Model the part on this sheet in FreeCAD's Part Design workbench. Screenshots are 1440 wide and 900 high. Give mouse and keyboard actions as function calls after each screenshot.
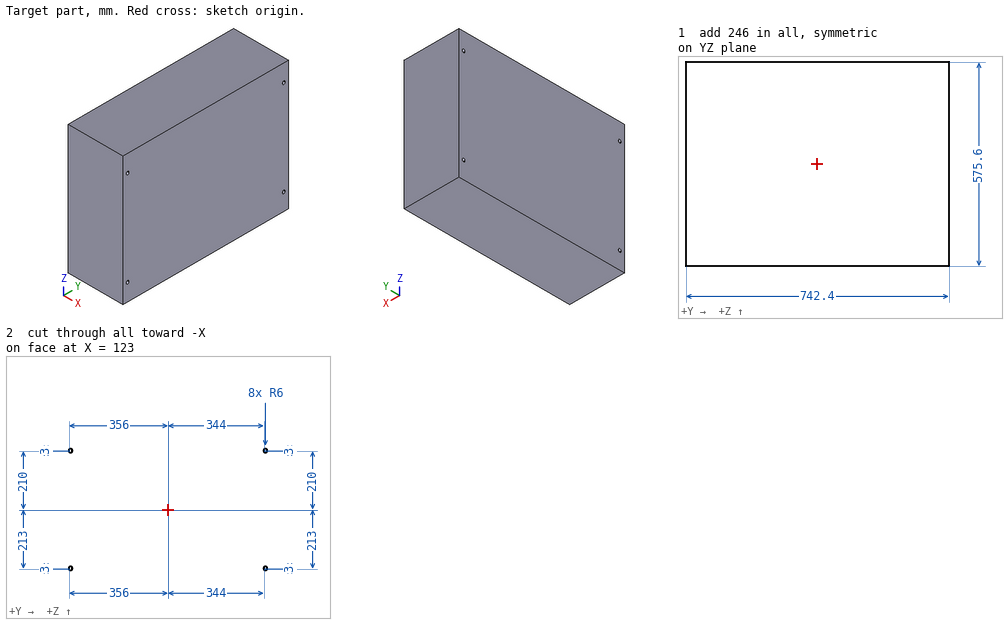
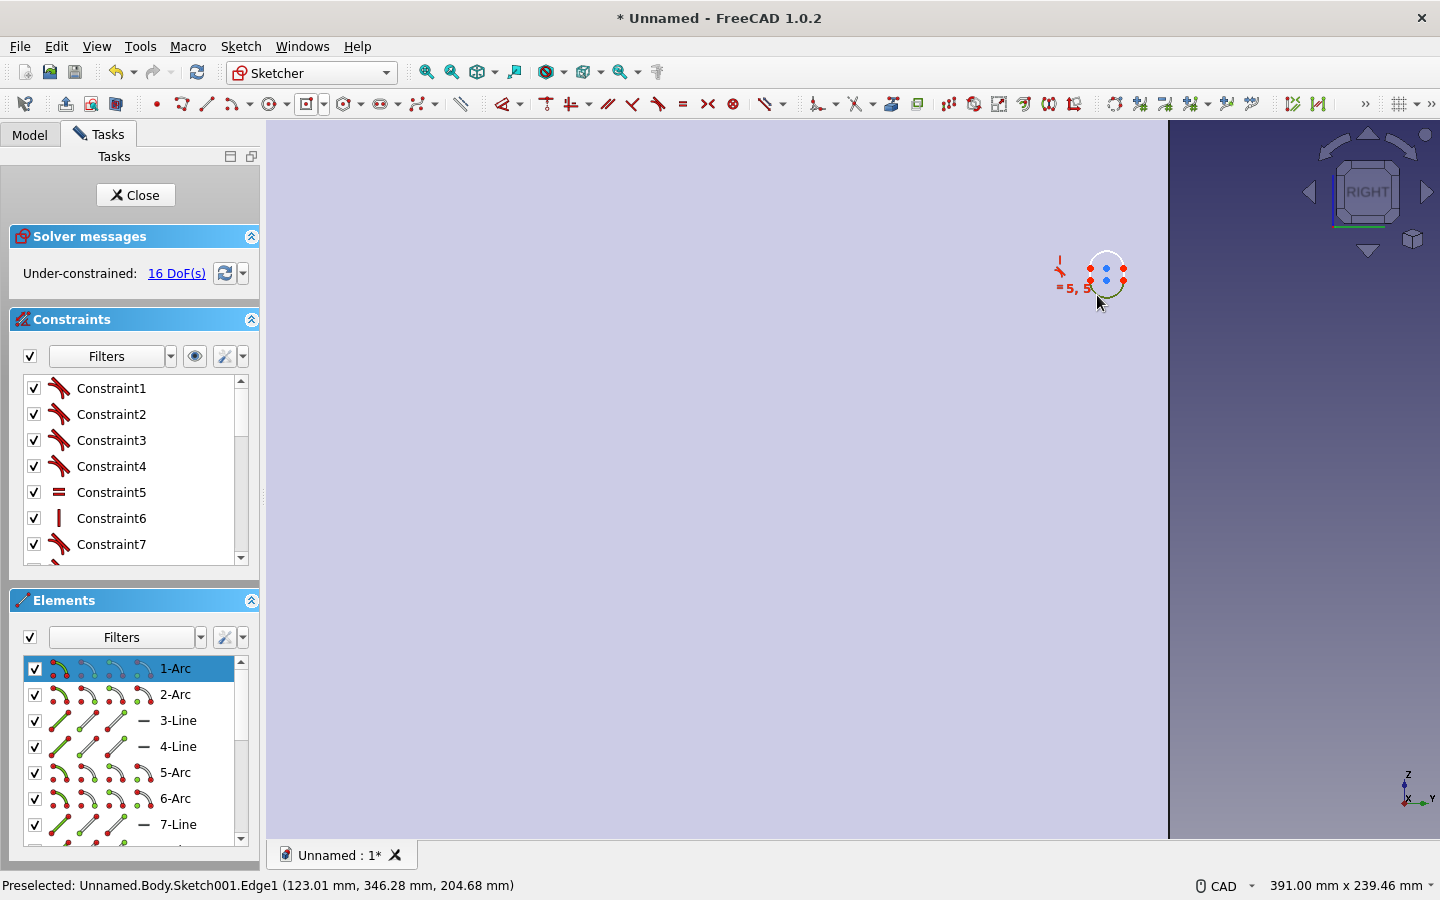
scroll(1099, 295, down, 6)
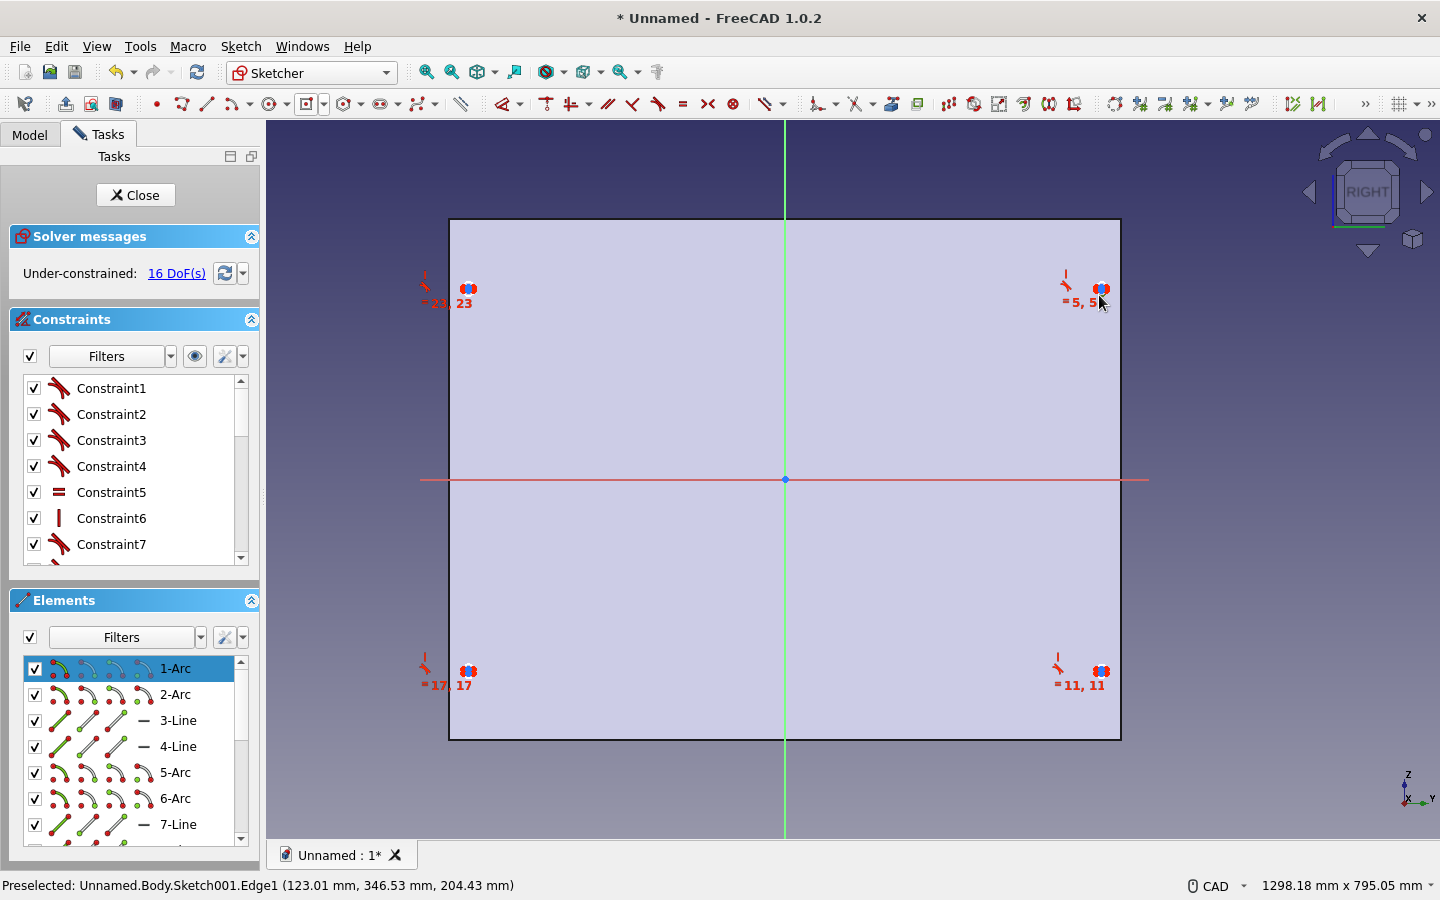
scroll(1099, 677, up, 6)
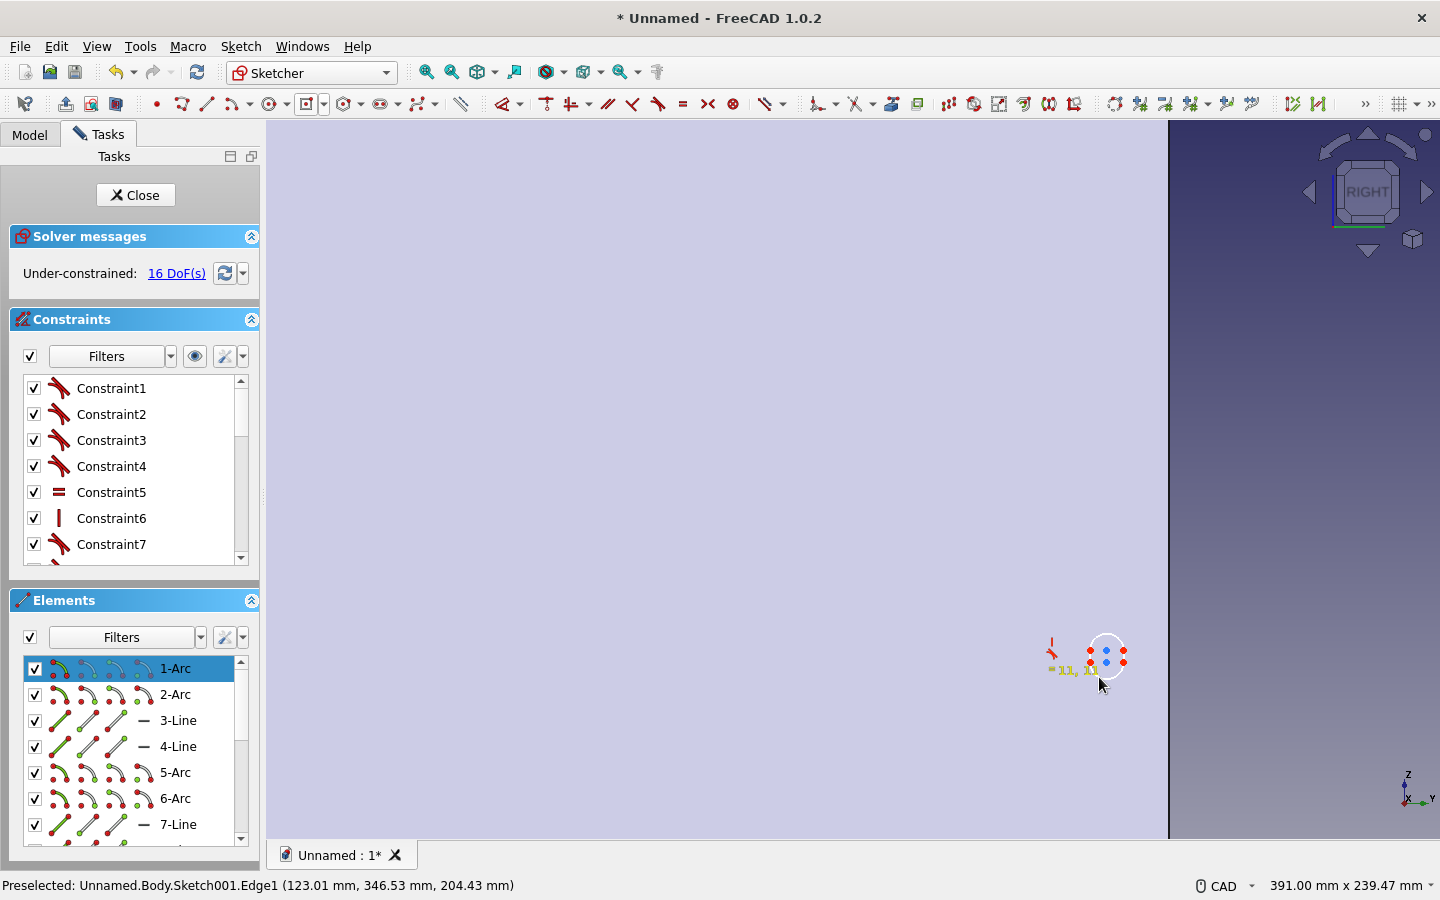
click(1097, 676)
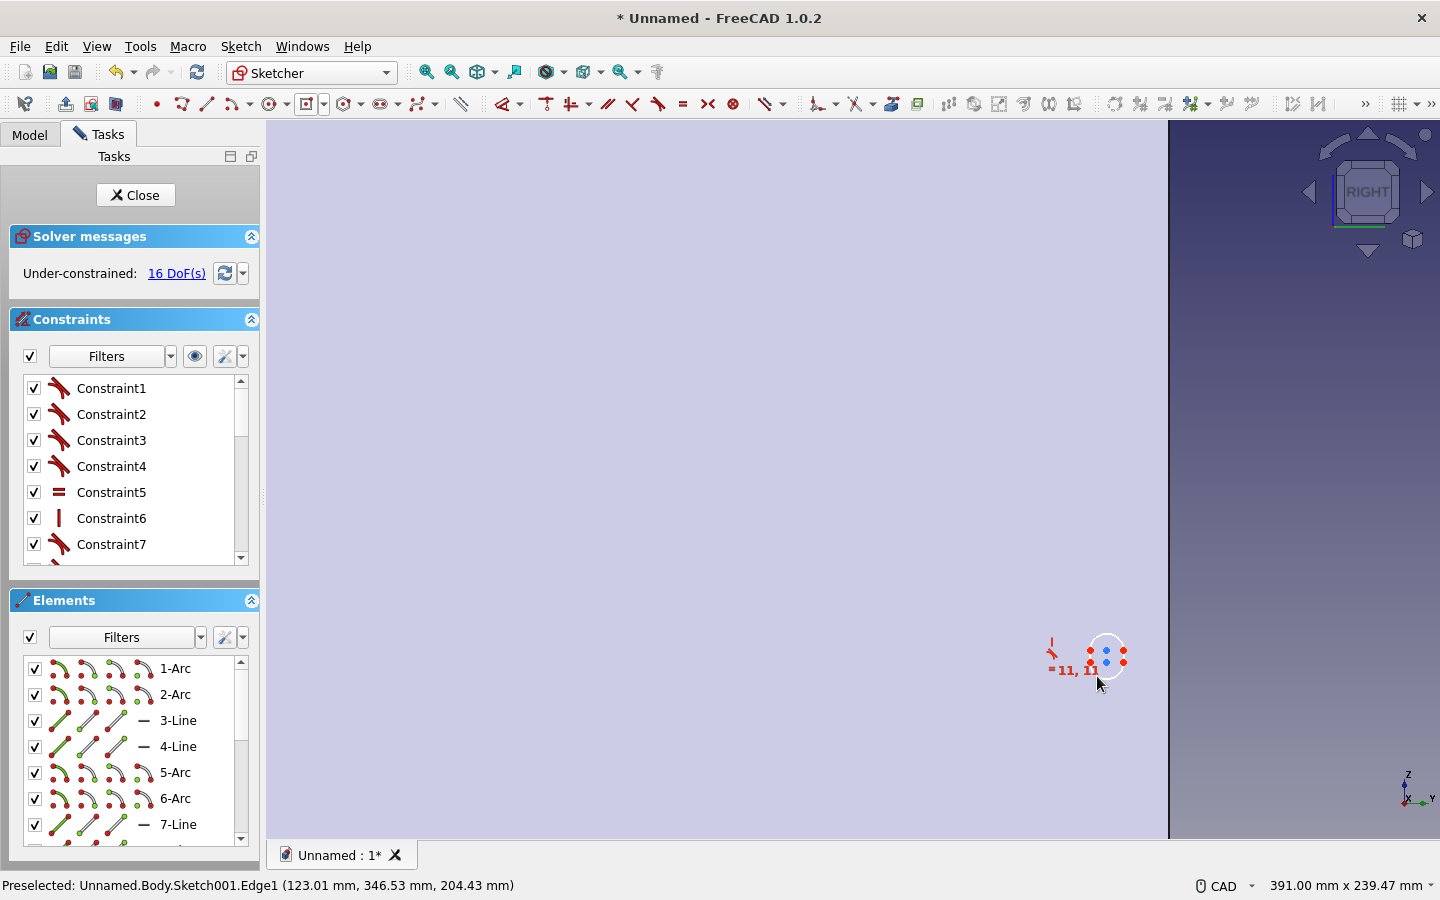
scroll(1099, 678, down, 6)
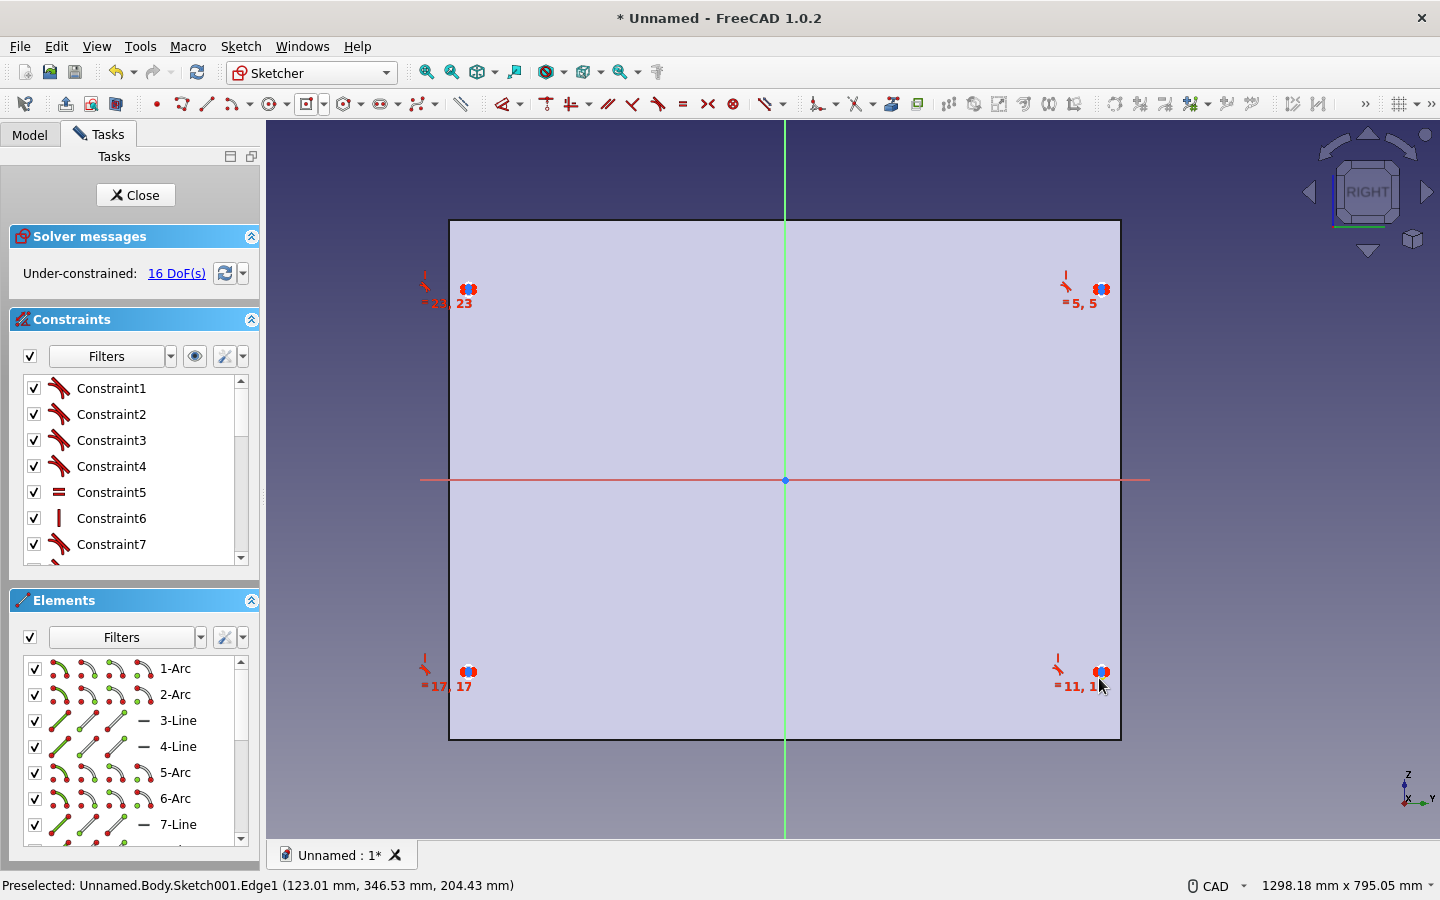
scroll(466, 678, up, 6)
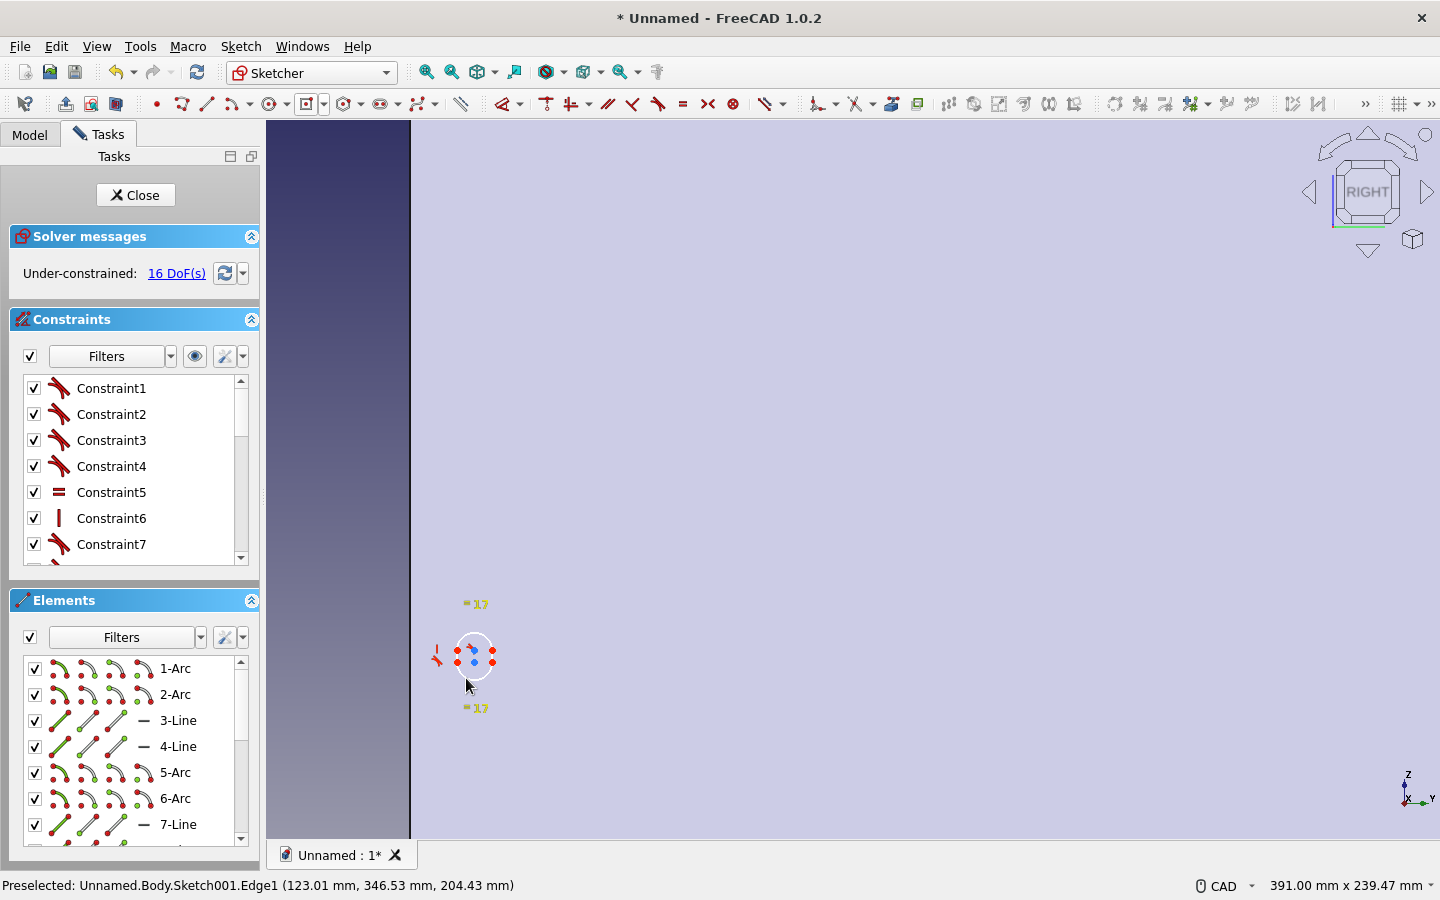
click(464, 677)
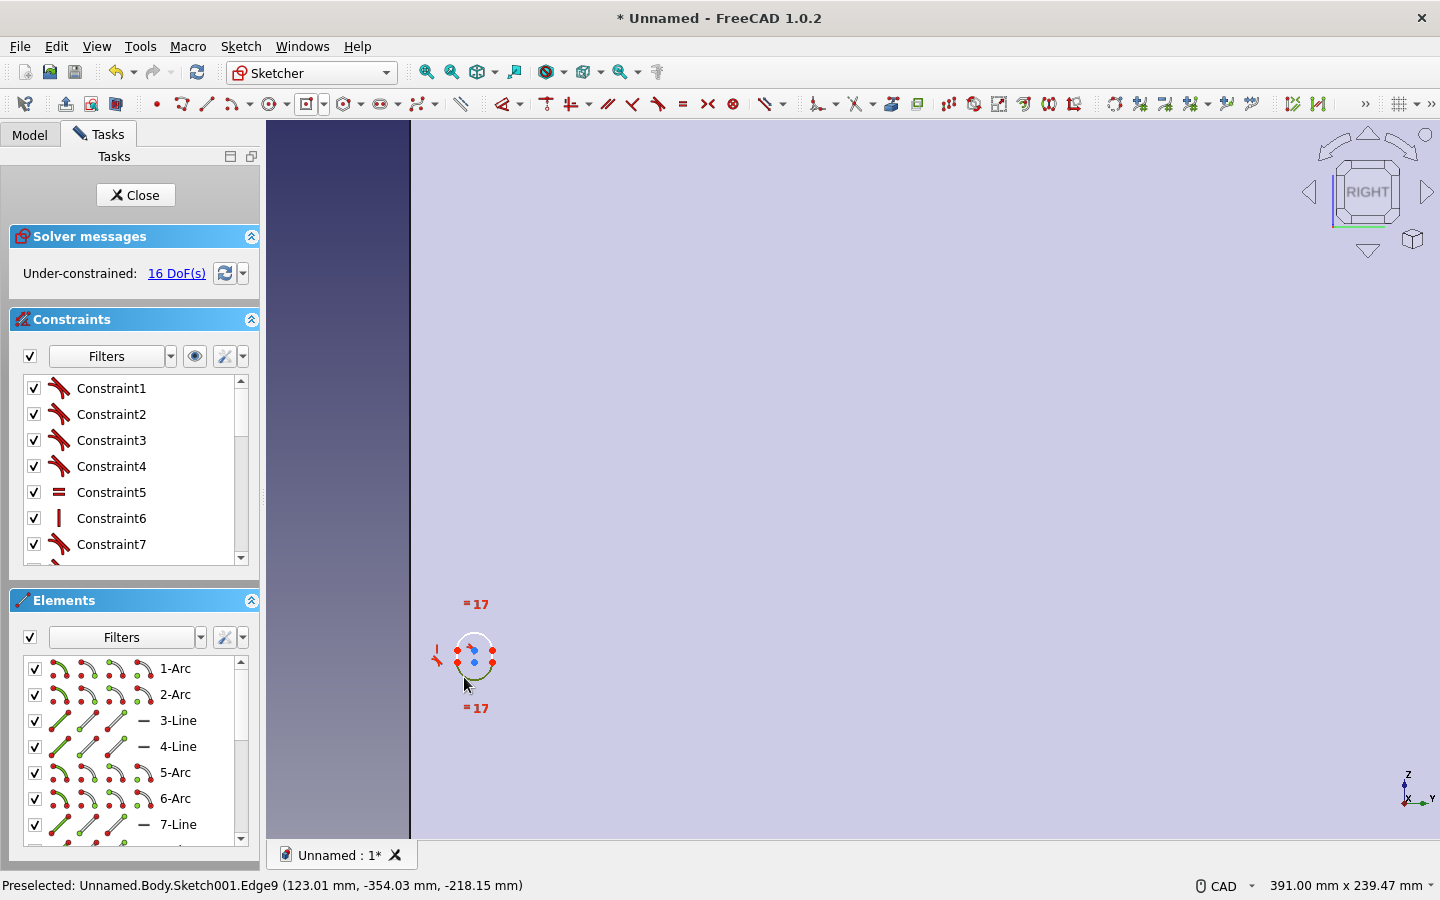
scroll(465, 678, down, 6)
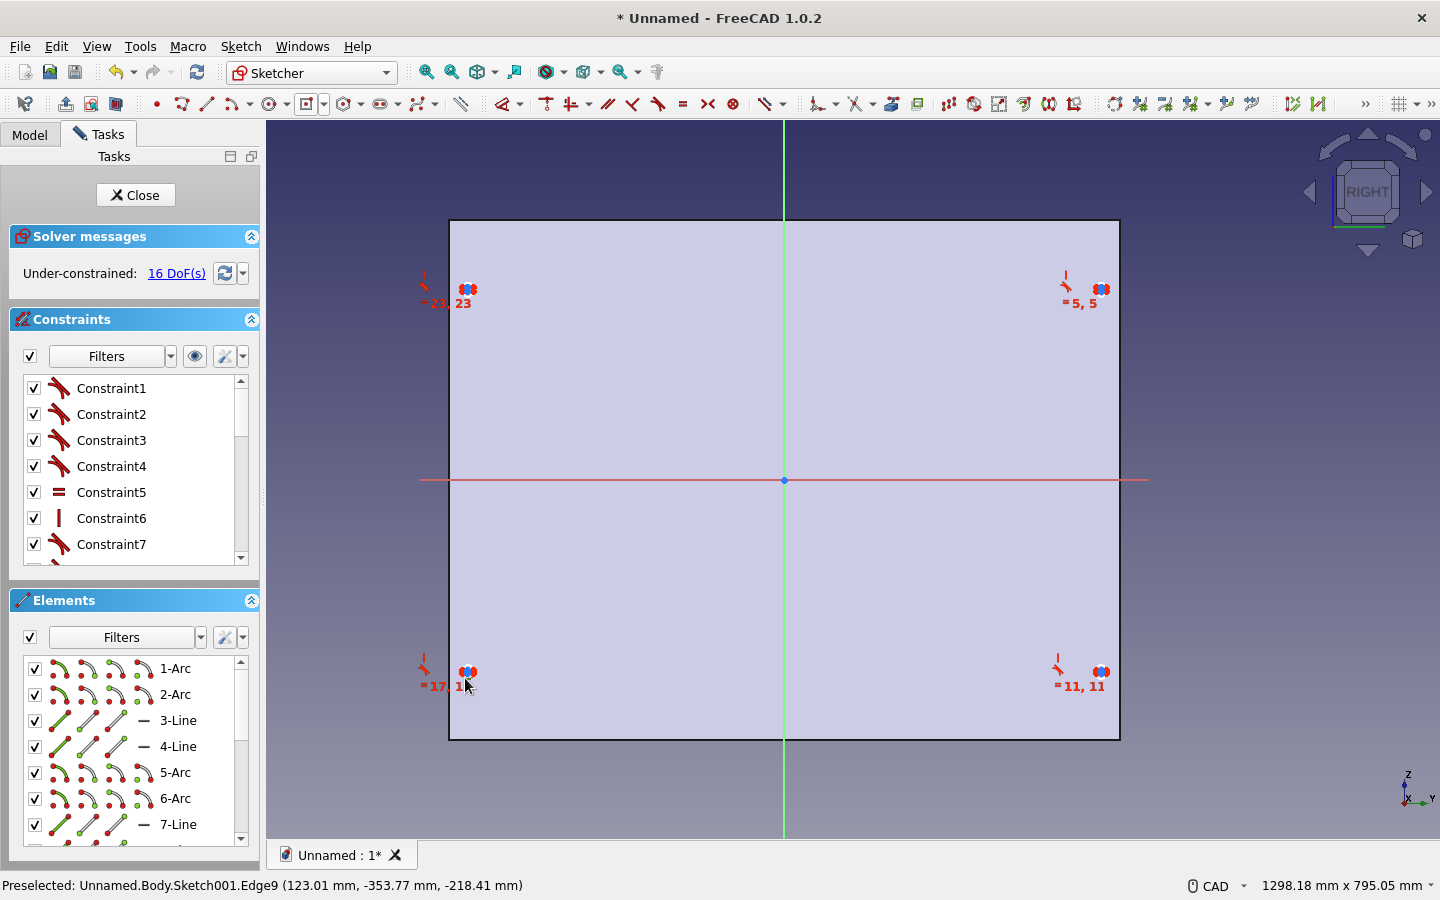
scroll(465, 296, up, 6)